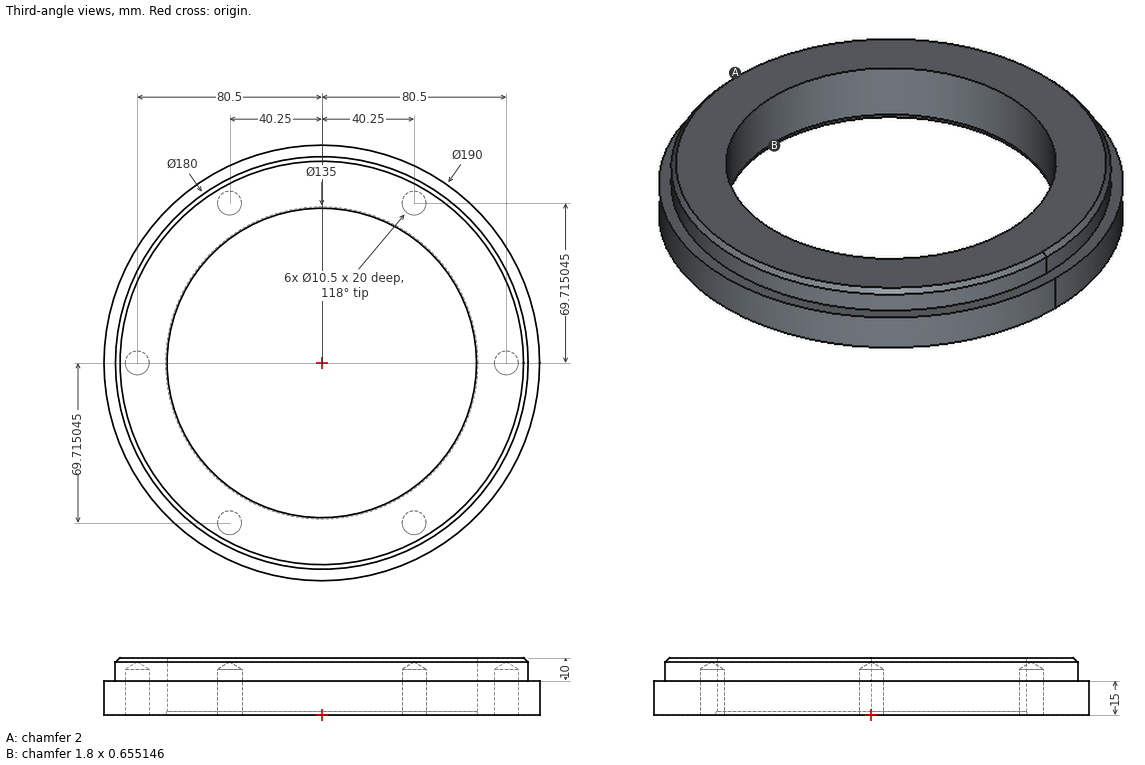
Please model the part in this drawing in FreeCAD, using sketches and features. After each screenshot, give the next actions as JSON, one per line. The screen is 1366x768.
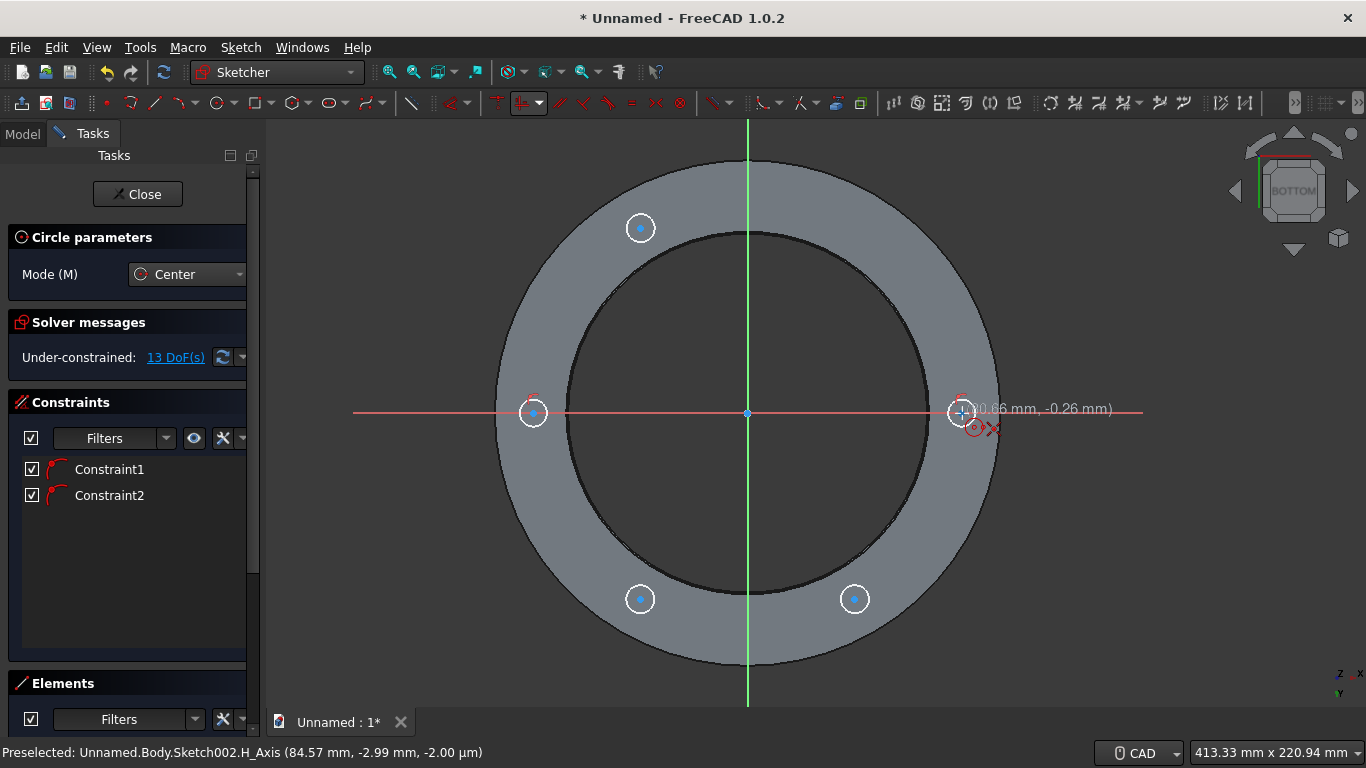
{"action": "scroll", "coordinate": [855, 228], "scroll_direction": "up", "scroll_amount": 3}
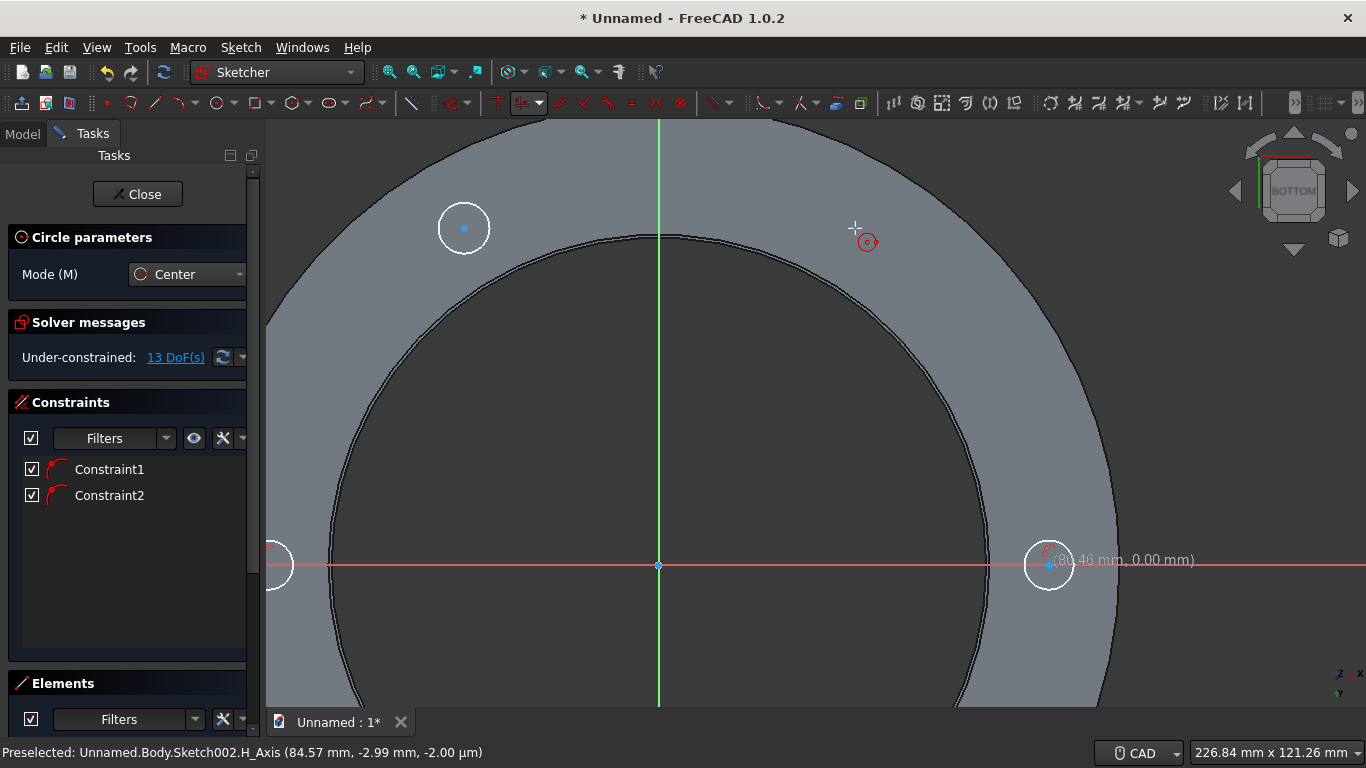
{"action": "left_click", "coordinate": [854, 227]}
{"action": "left_click", "coordinate": [872, 209]}
{"action": "key", "text": "Escape"}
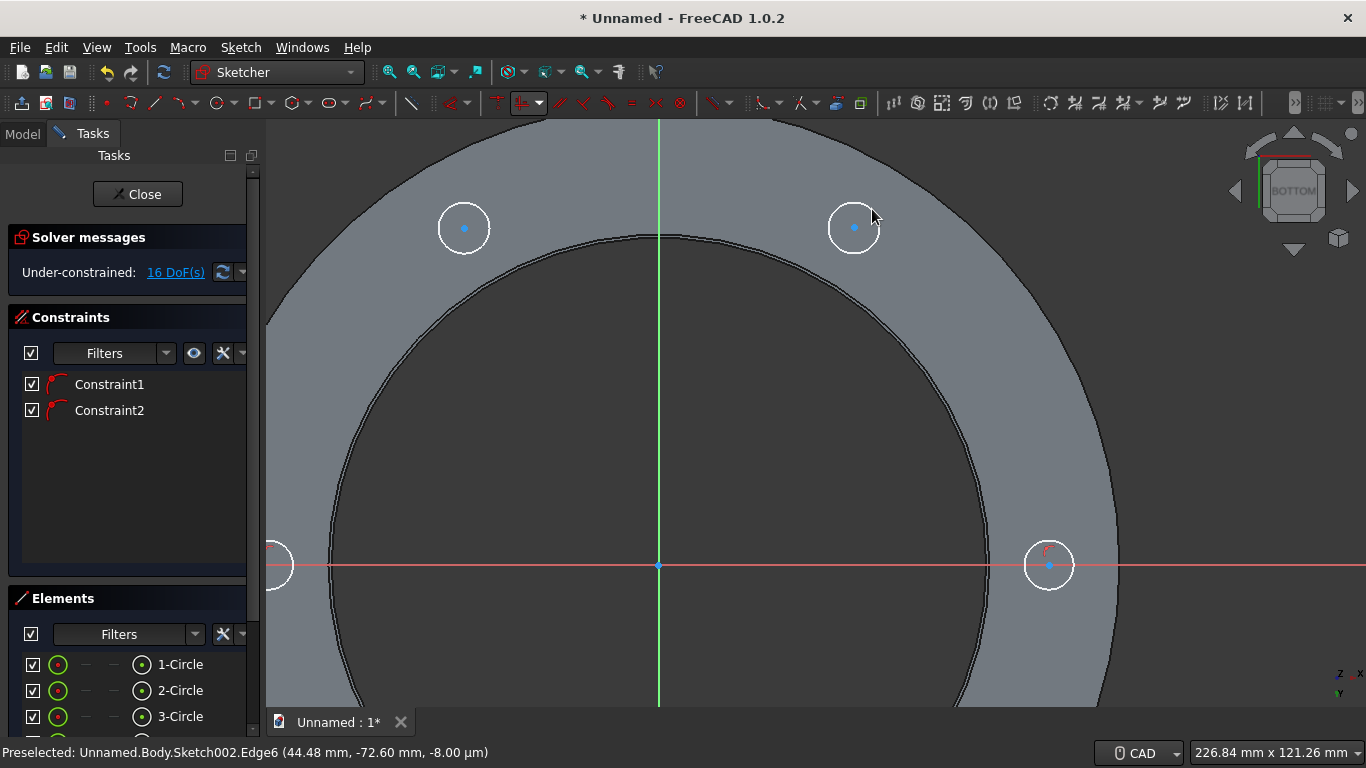
{"action": "scroll", "coordinate": [855, 228], "scroll_direction": "down", "scroll_amount": 3}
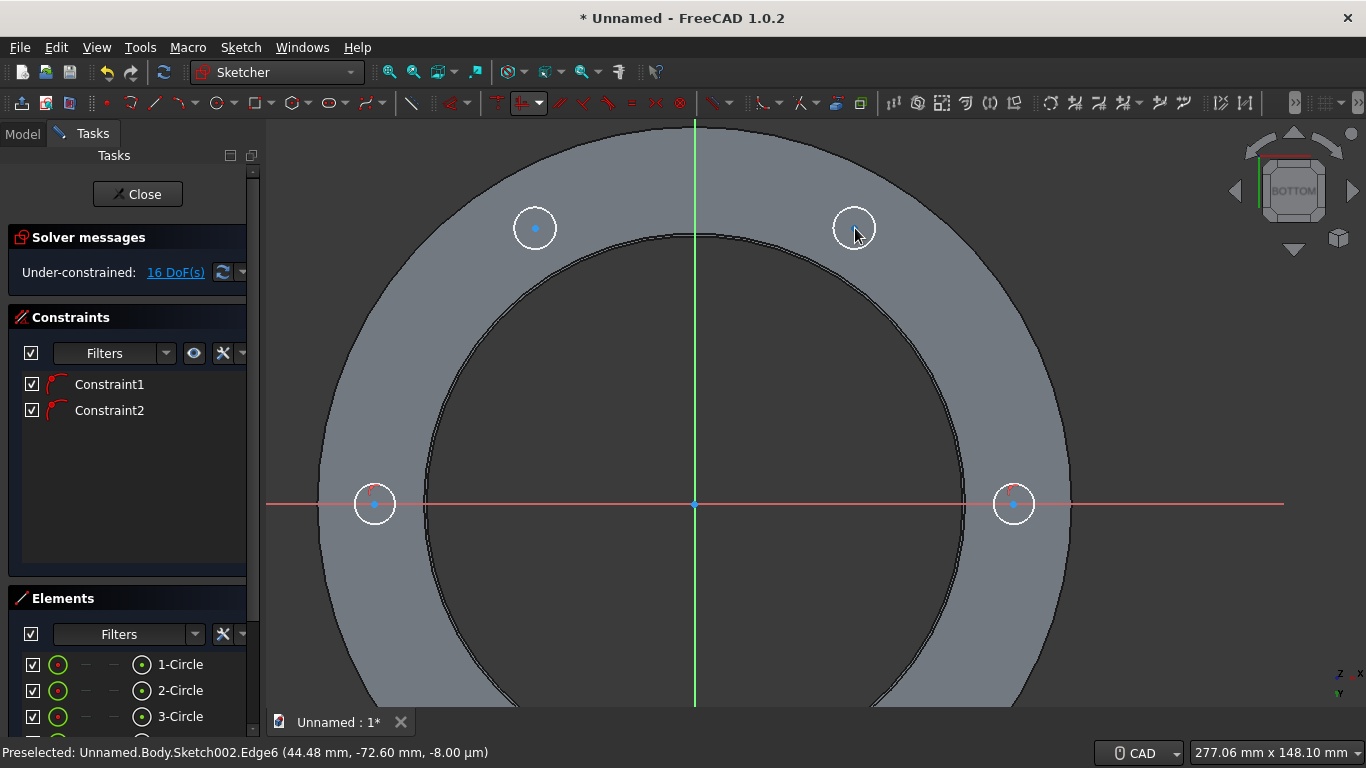
{"action": "left_click", "coordinate": [865, 589]}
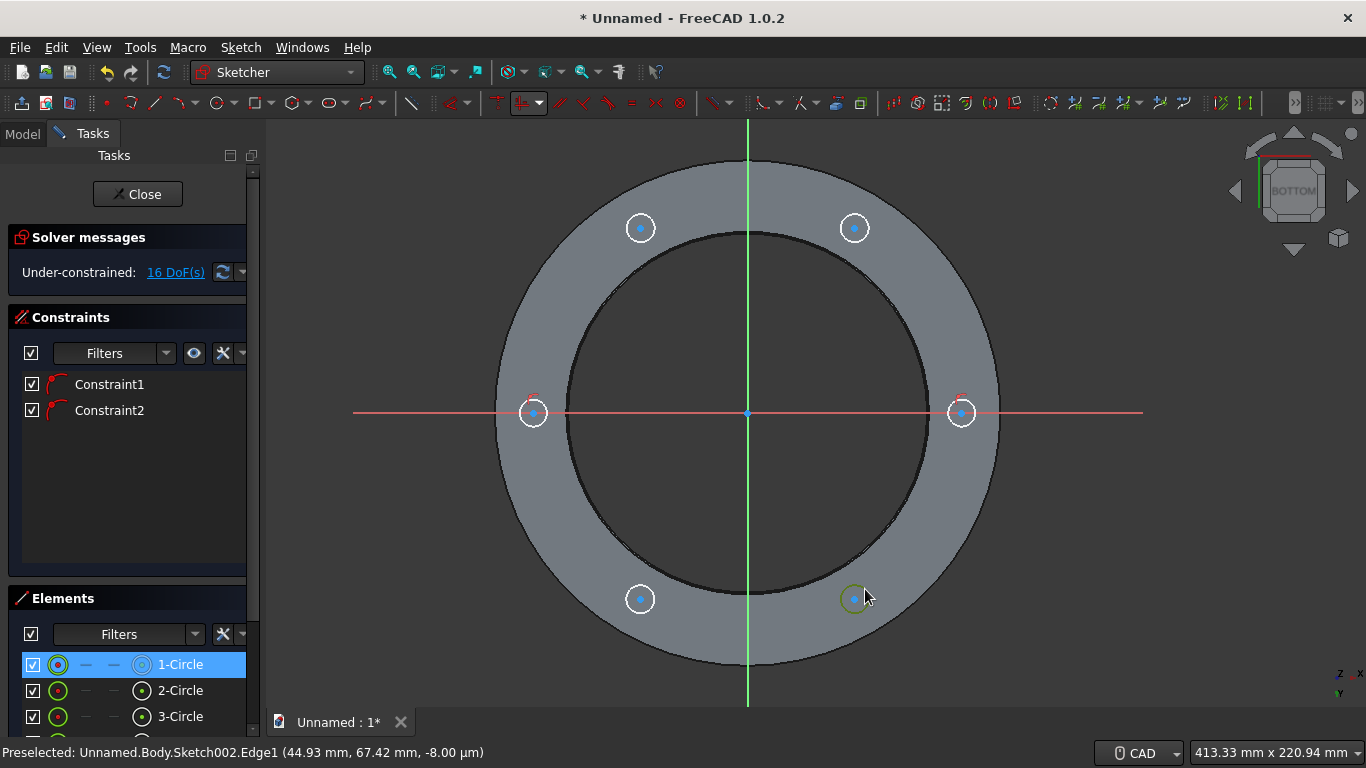
{"action": "left_click", "coordinate": [650, 589]}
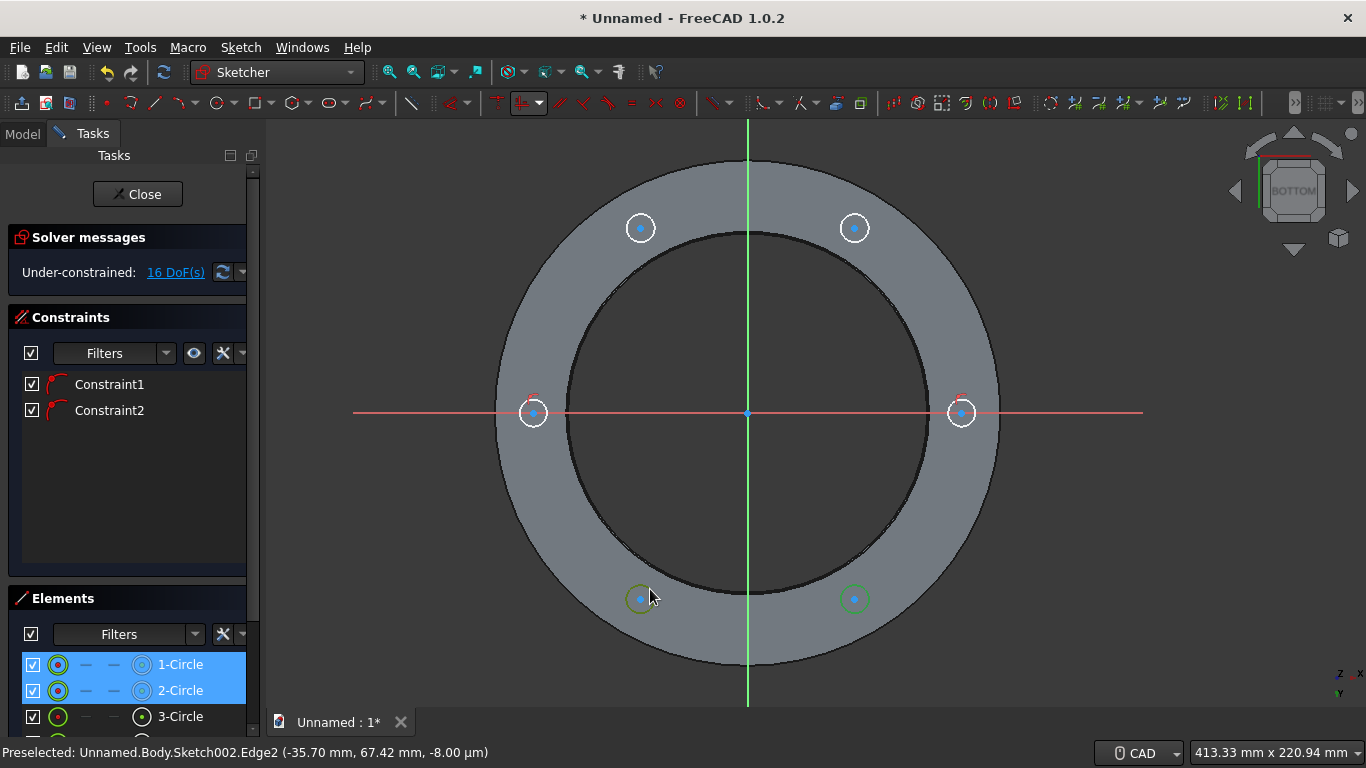
{"action": "scroll", "coordinate": [543, 403], "scroll_direction": "up", "scroll_amount": 2}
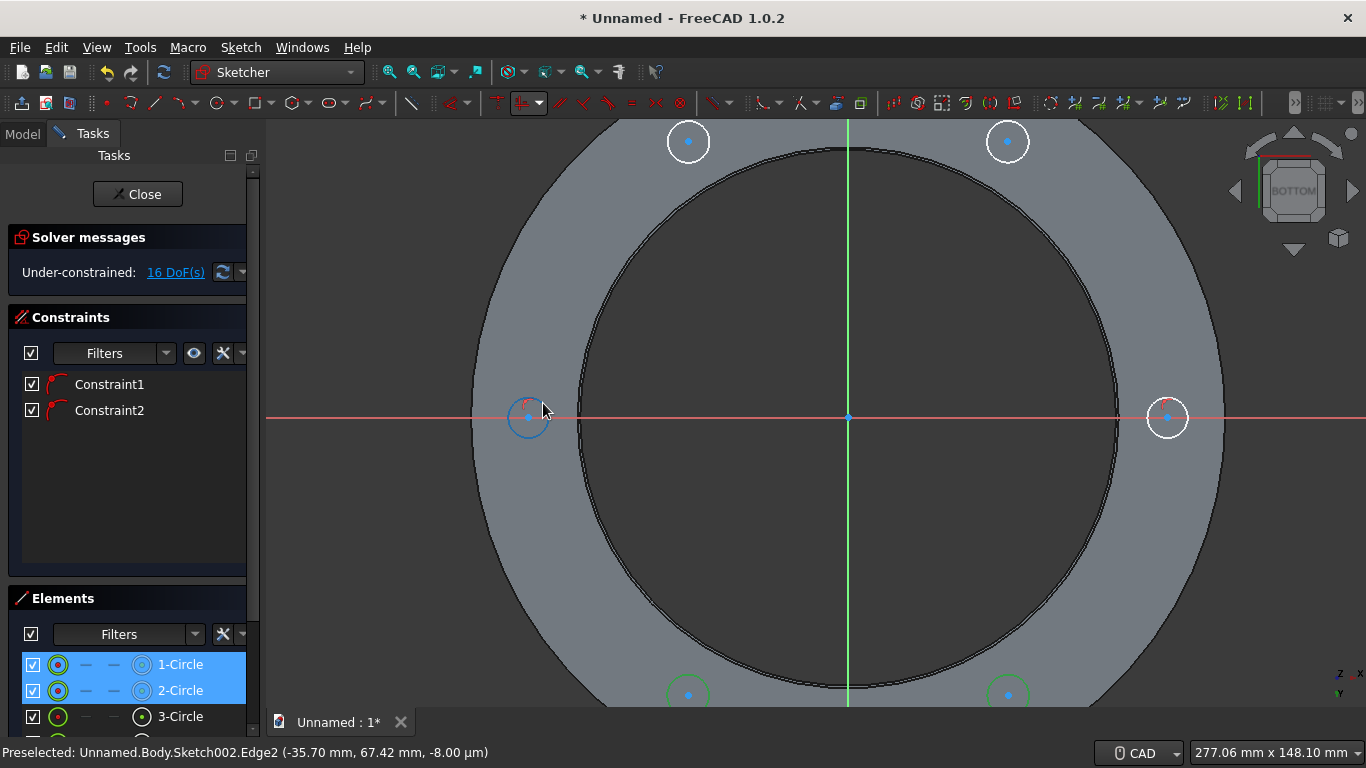
{"action": "left_click", "coordinate": [543, 403]}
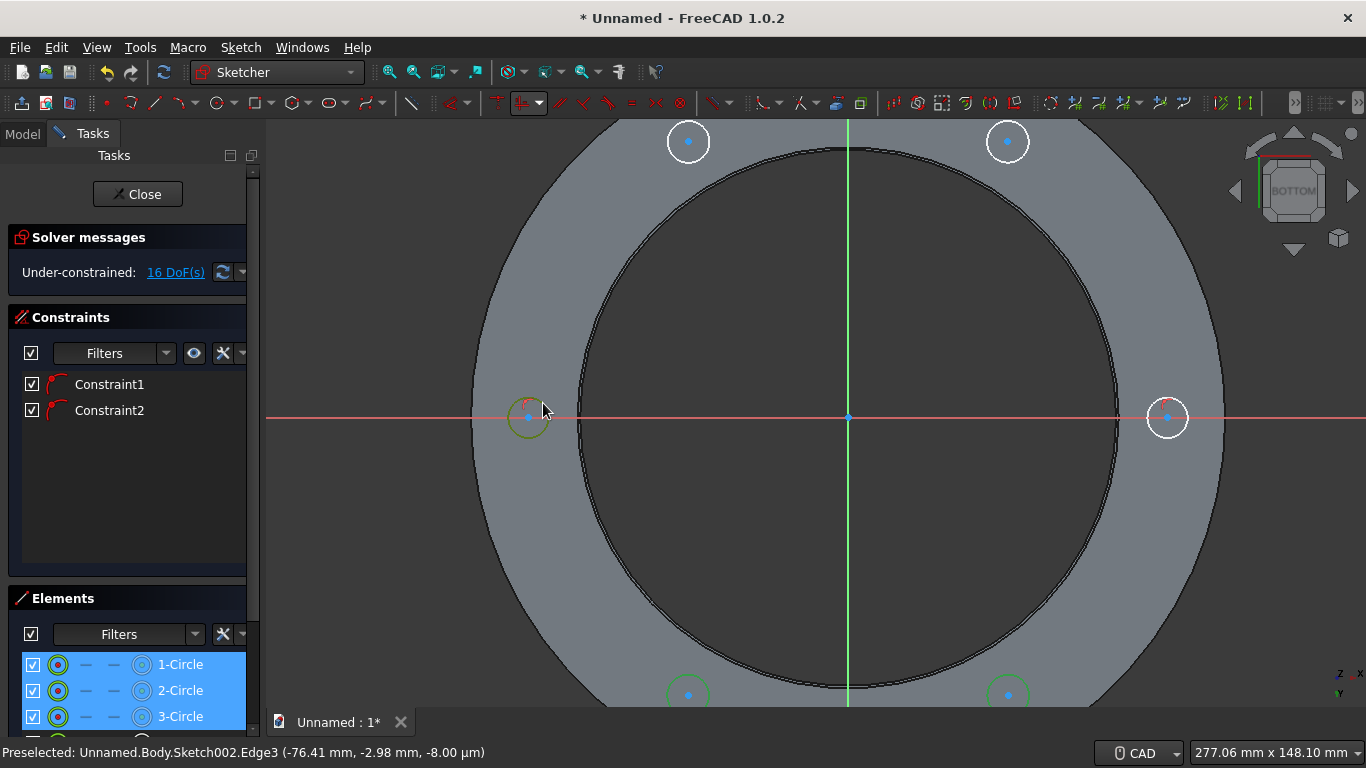
{"action": "left_click", "coordinate": [674, 157]}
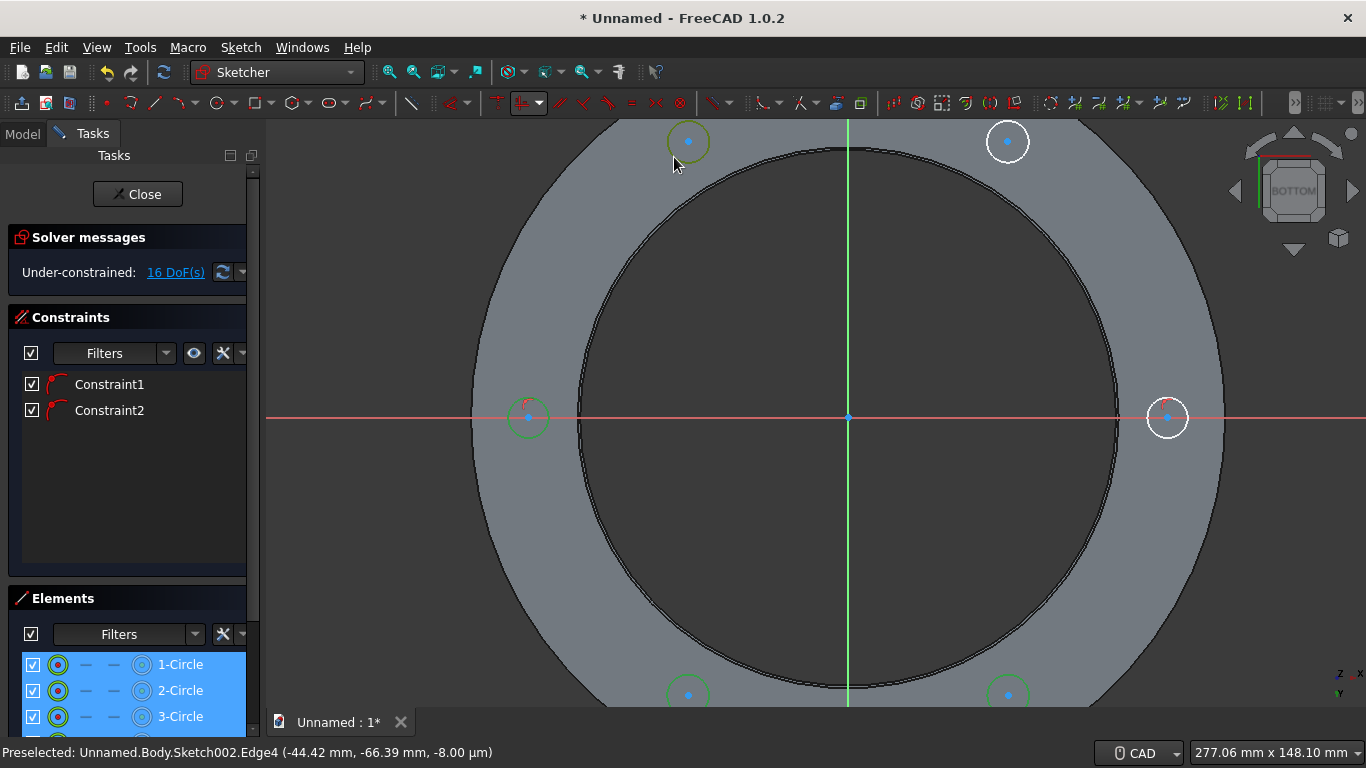
{"action": "left_click", "coordinate": [1182, 404]}